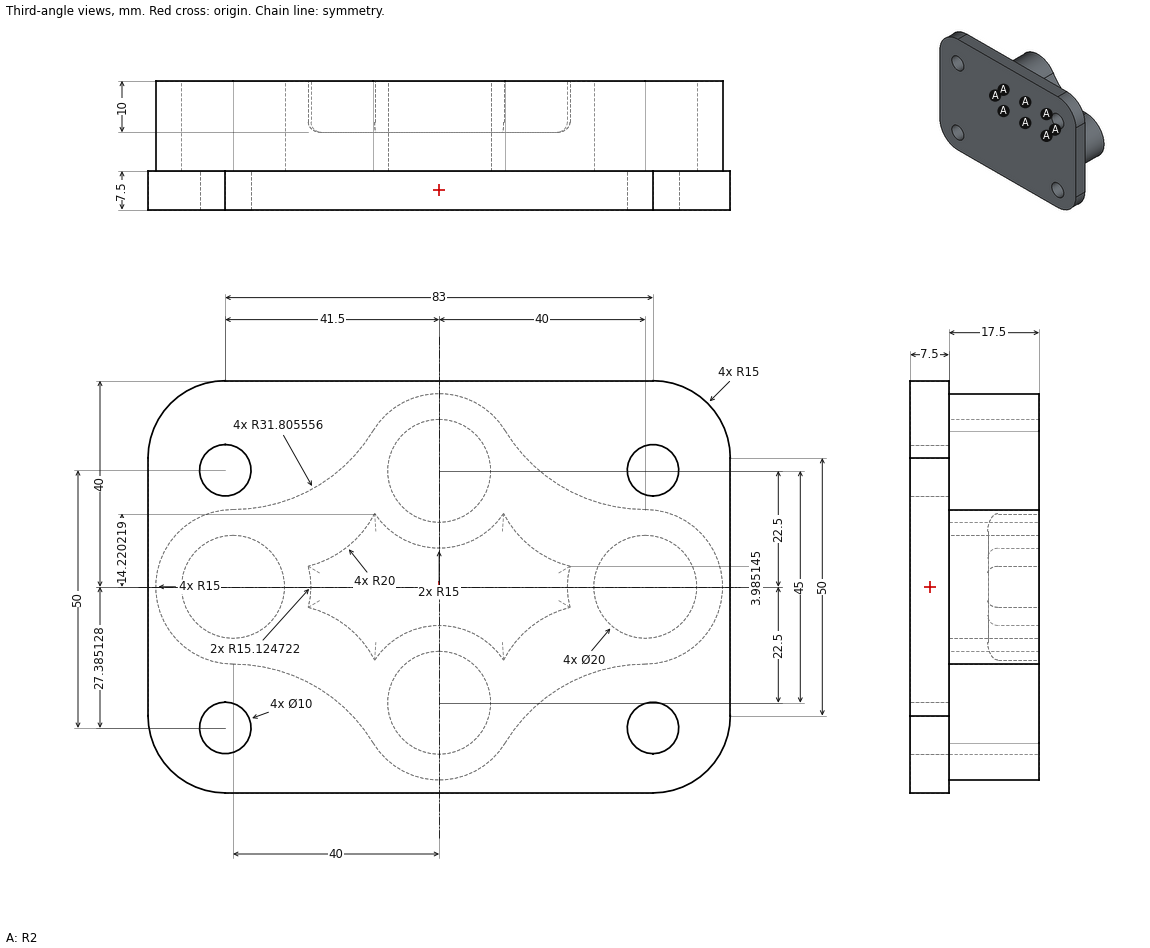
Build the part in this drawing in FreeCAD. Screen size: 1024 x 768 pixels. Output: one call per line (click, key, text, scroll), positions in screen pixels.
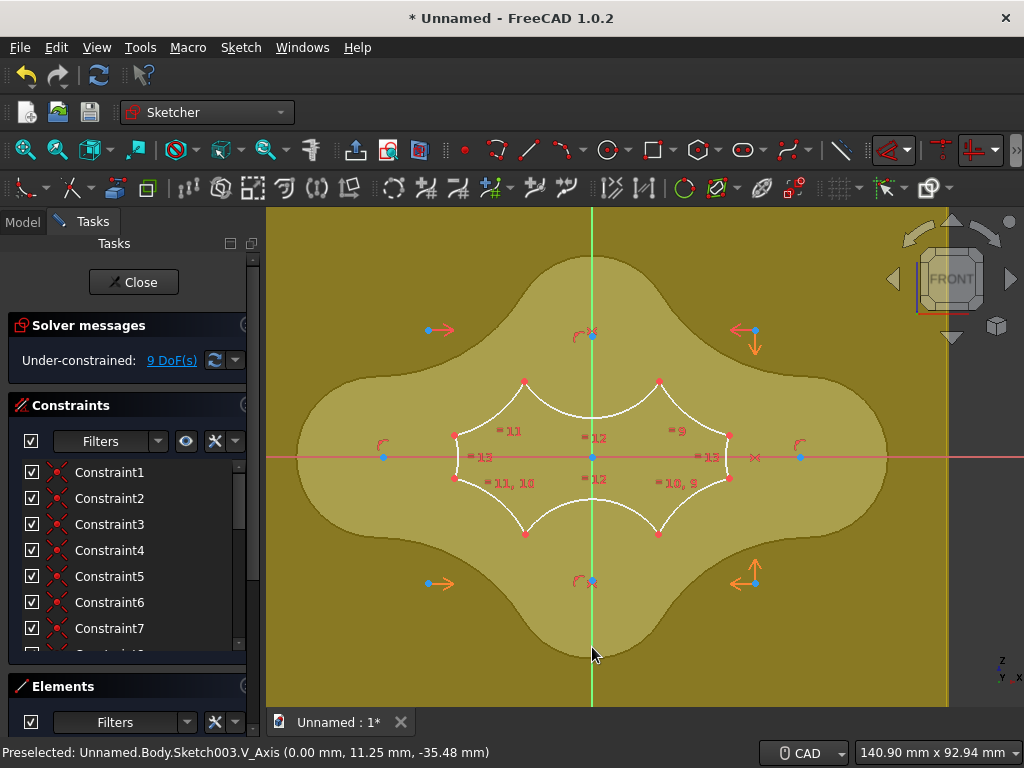
click(561, 412)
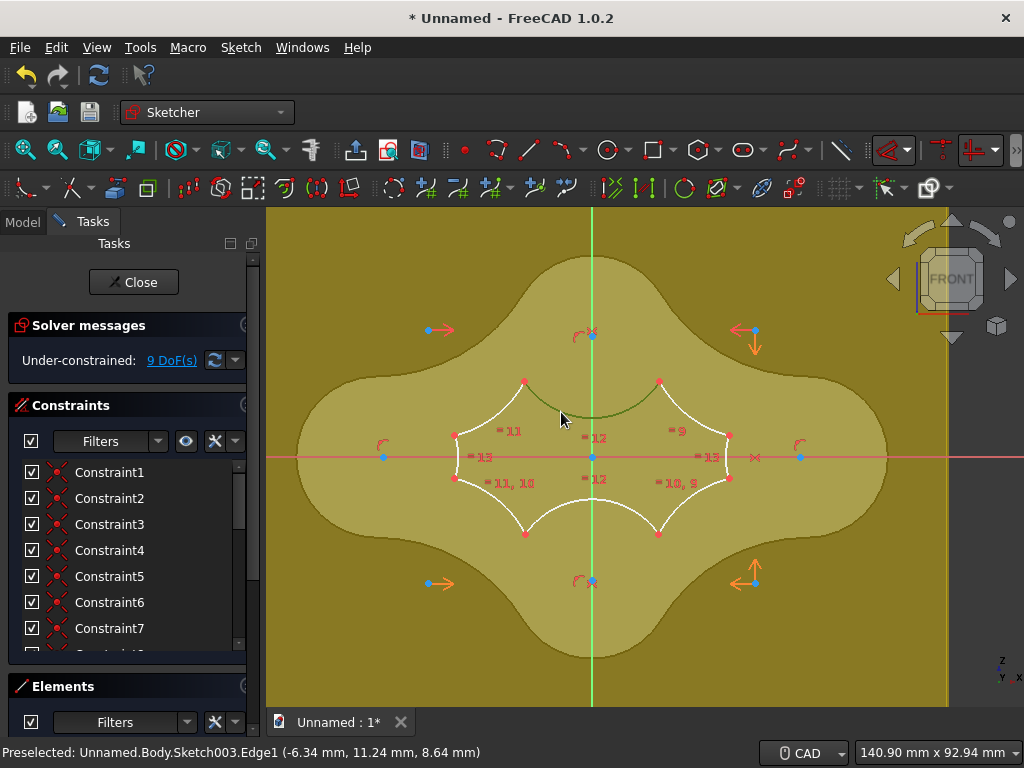
key(k)
key(r)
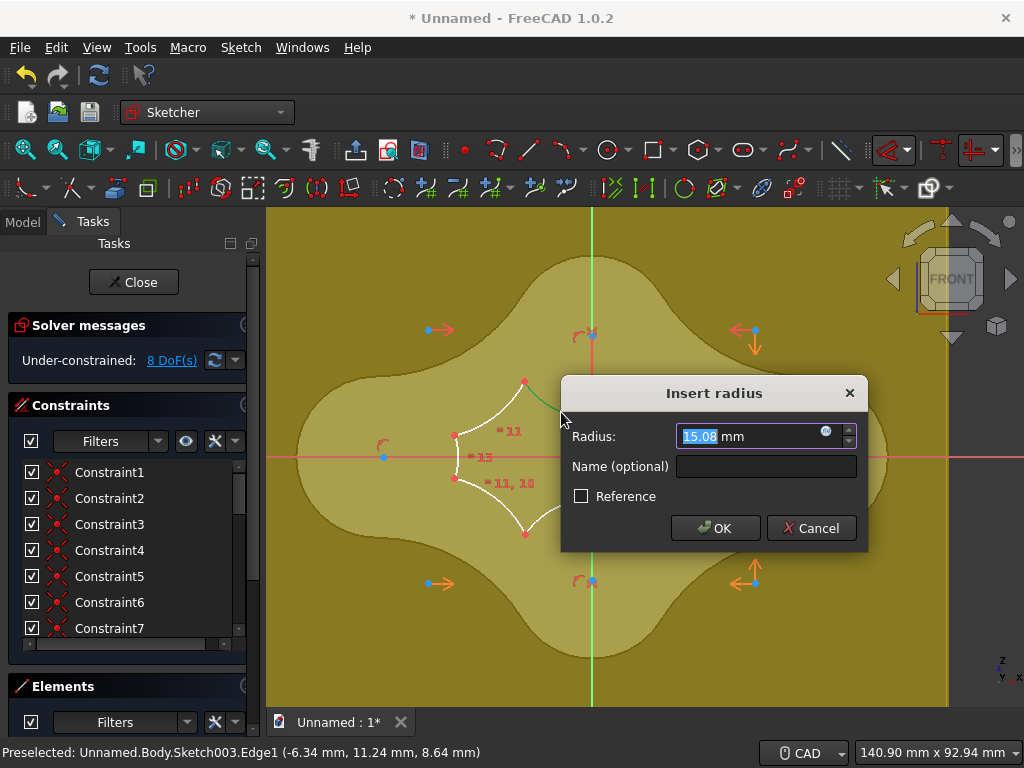
text(15)
key(Return)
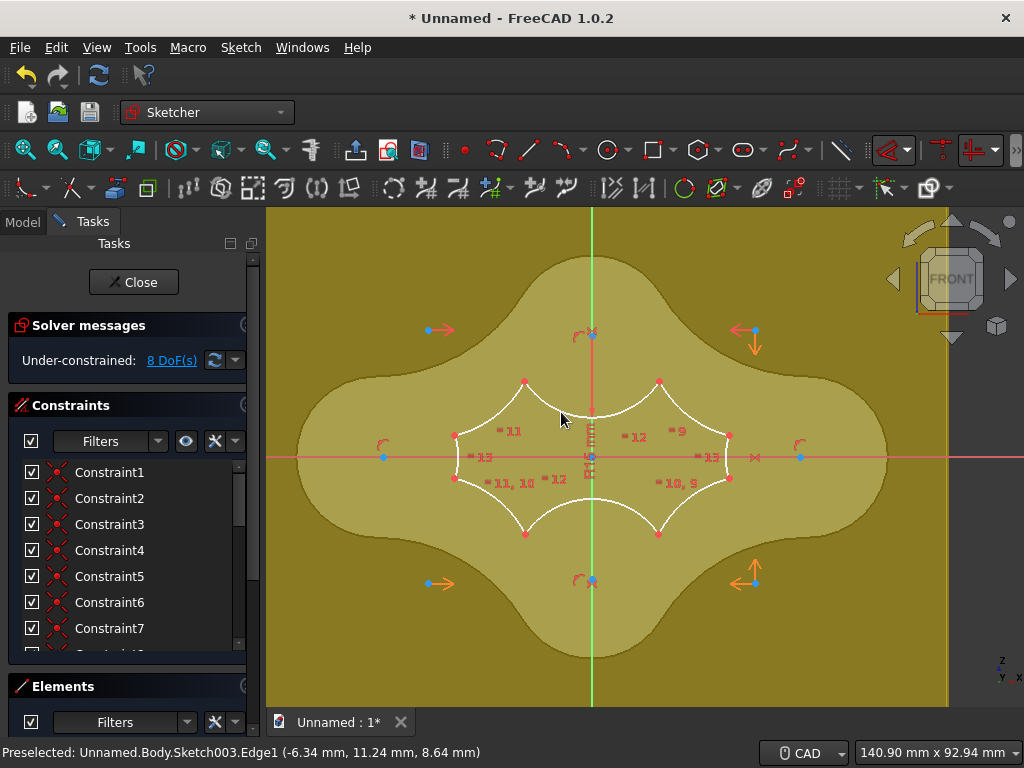
click(675, 404)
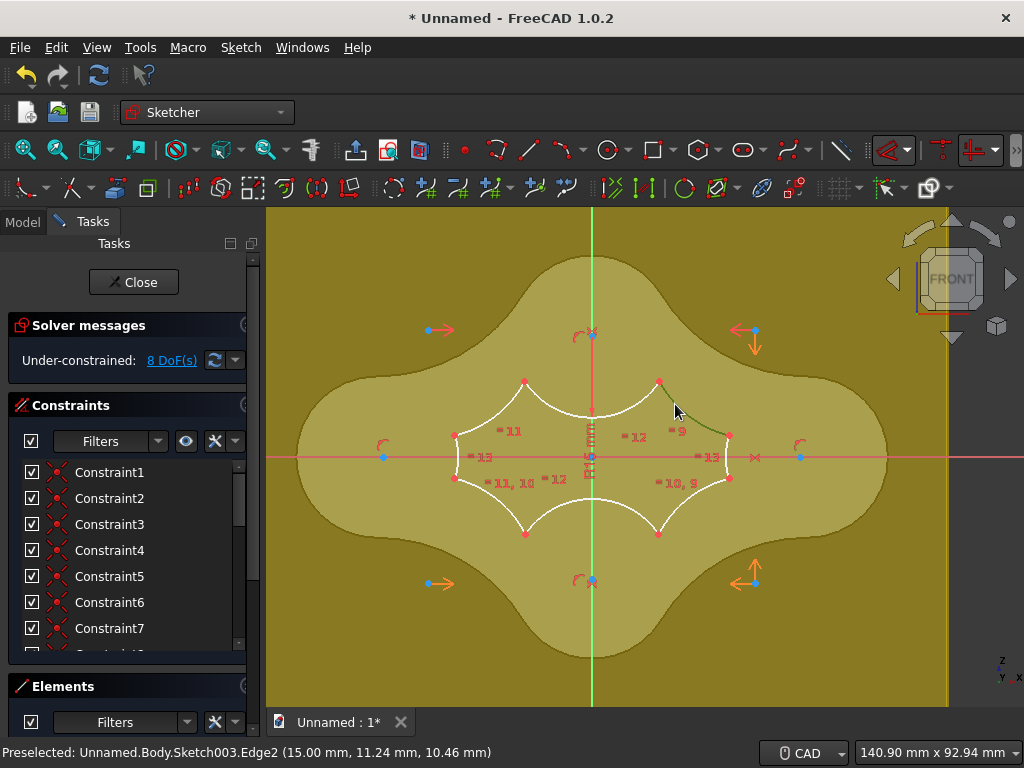
click(910, 150)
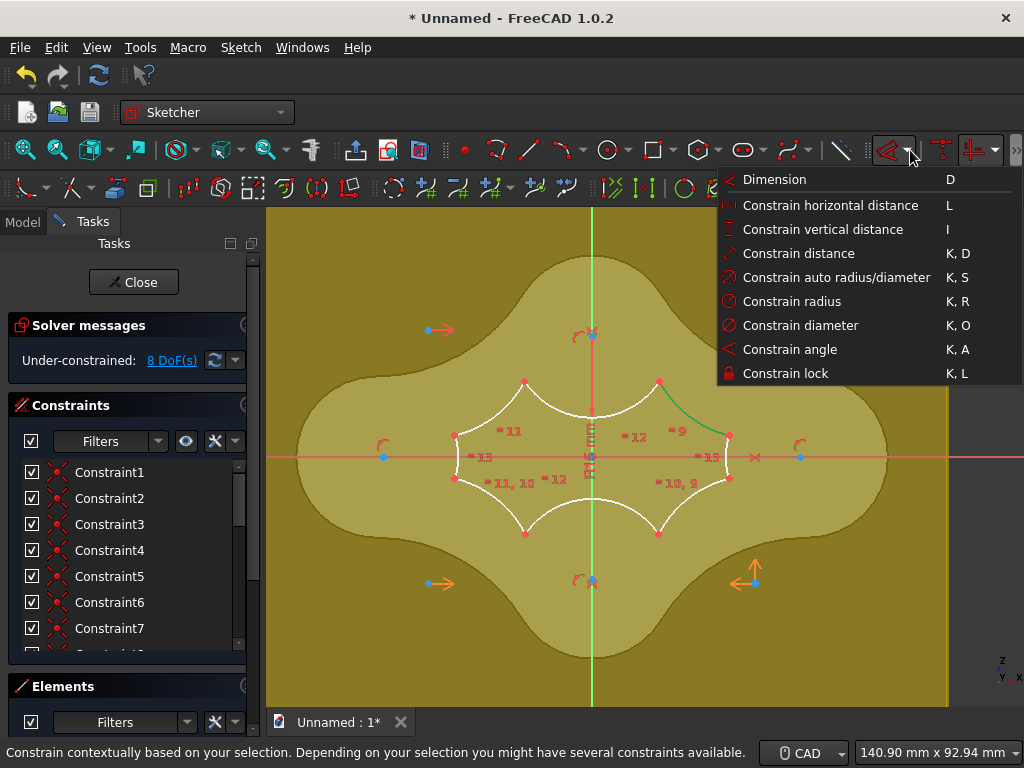
click(870, 301)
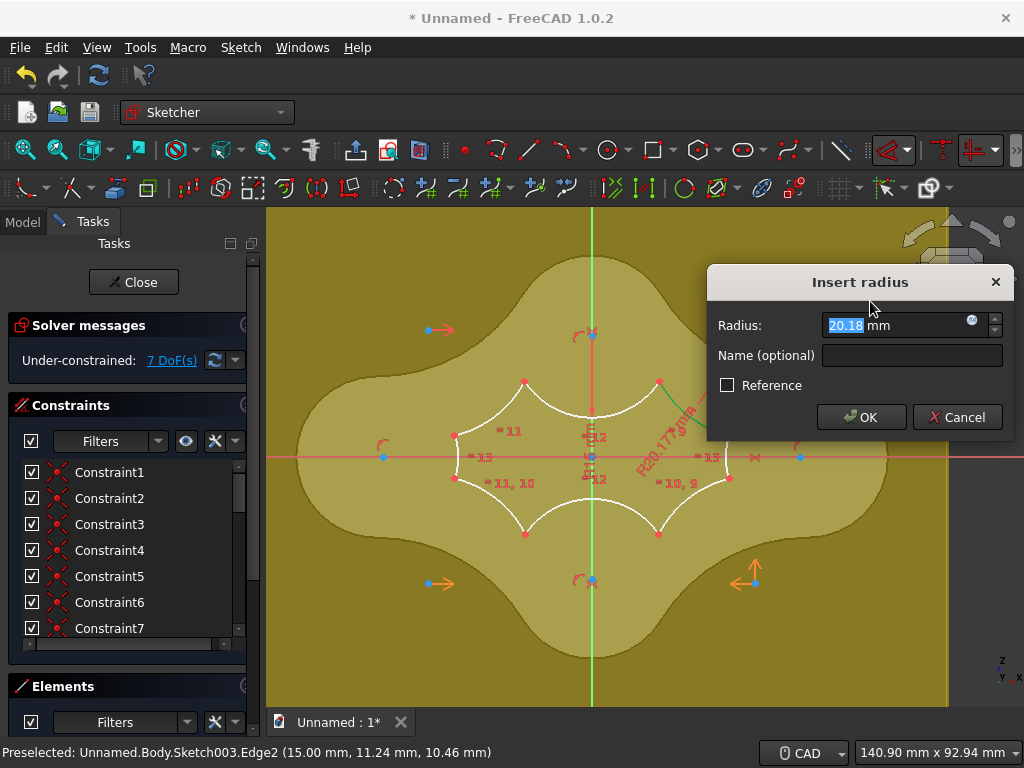
text(20)
key(Return)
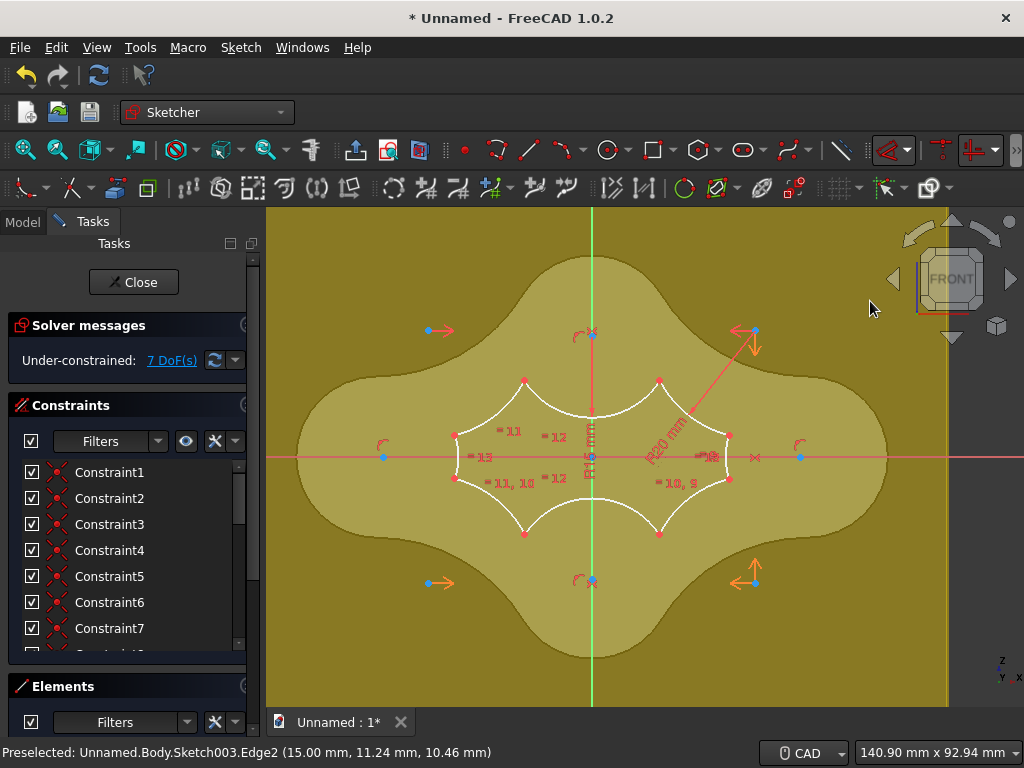
click(726, 457)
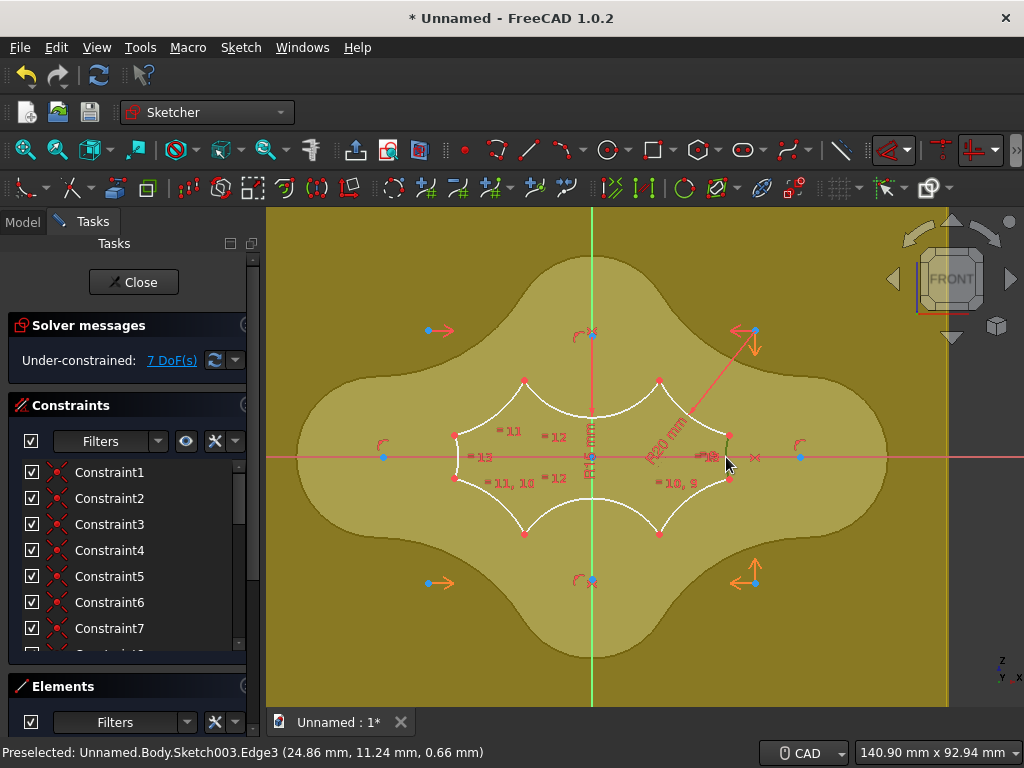
click(910, 150)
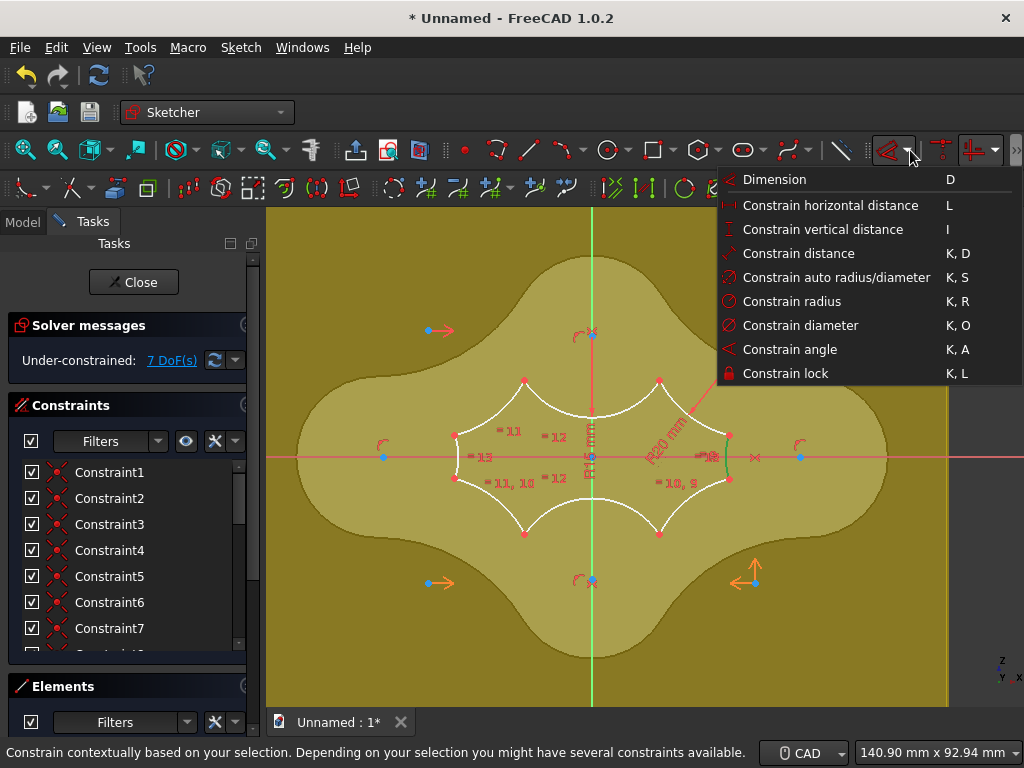
click(870, 301)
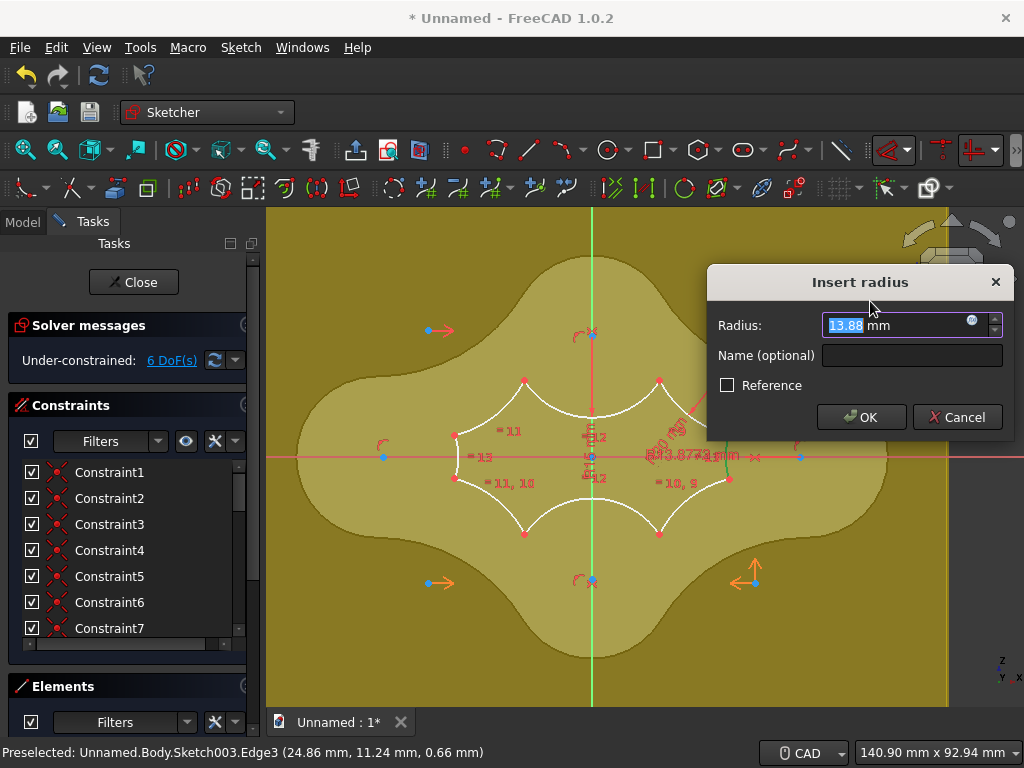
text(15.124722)
key(Return)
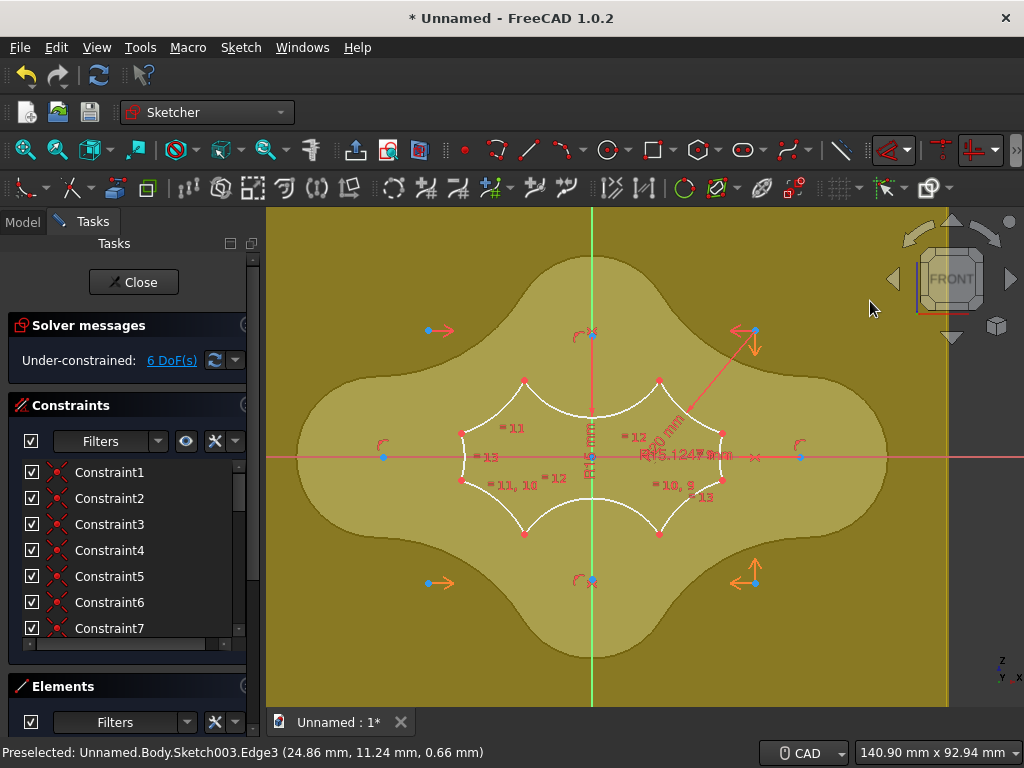
click(801, 457)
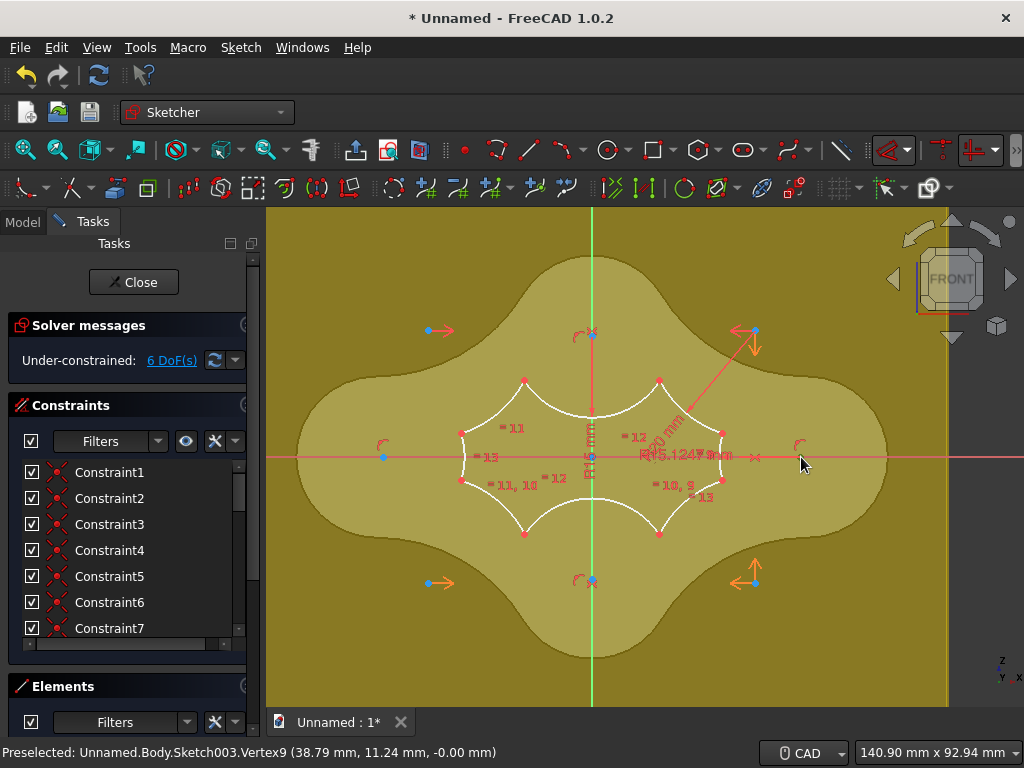
key(l)